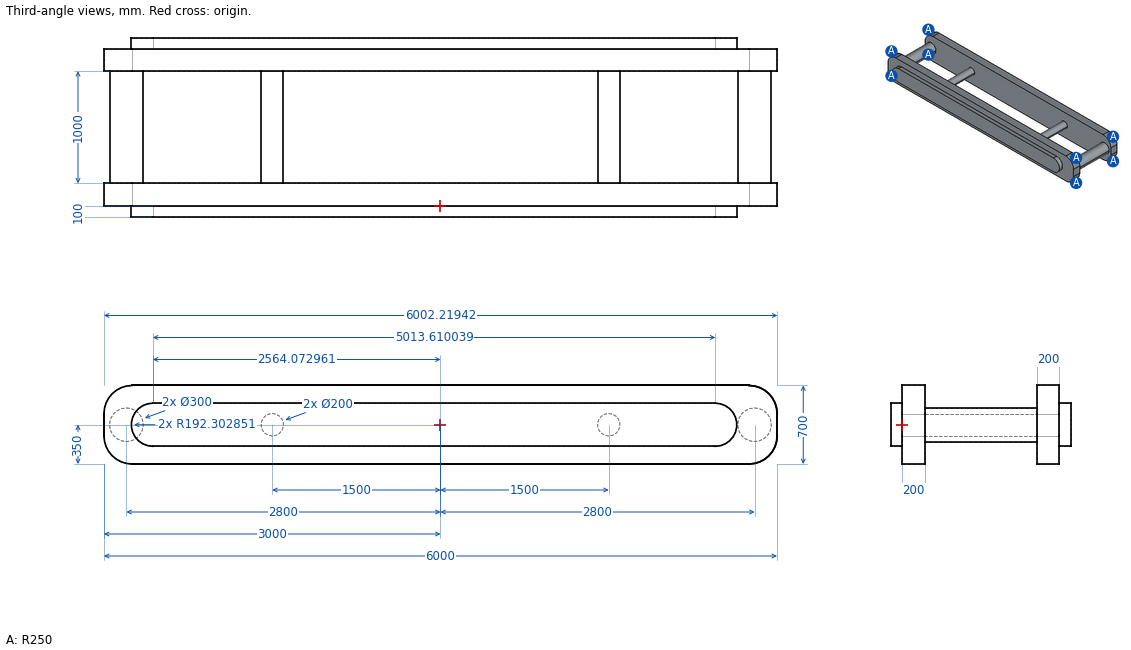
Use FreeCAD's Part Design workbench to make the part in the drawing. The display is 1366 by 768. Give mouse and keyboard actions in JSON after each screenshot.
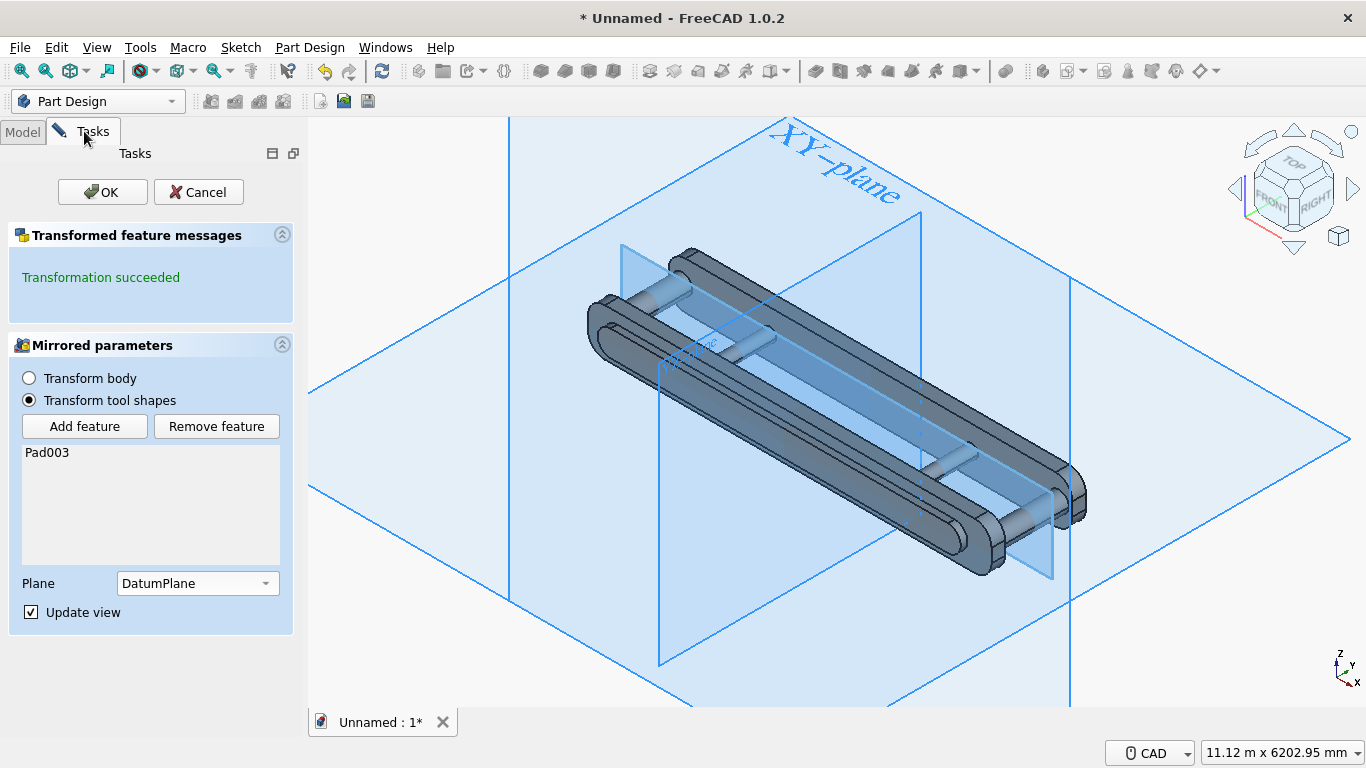
{"action": "left_click", "coordinate": [103, 192]}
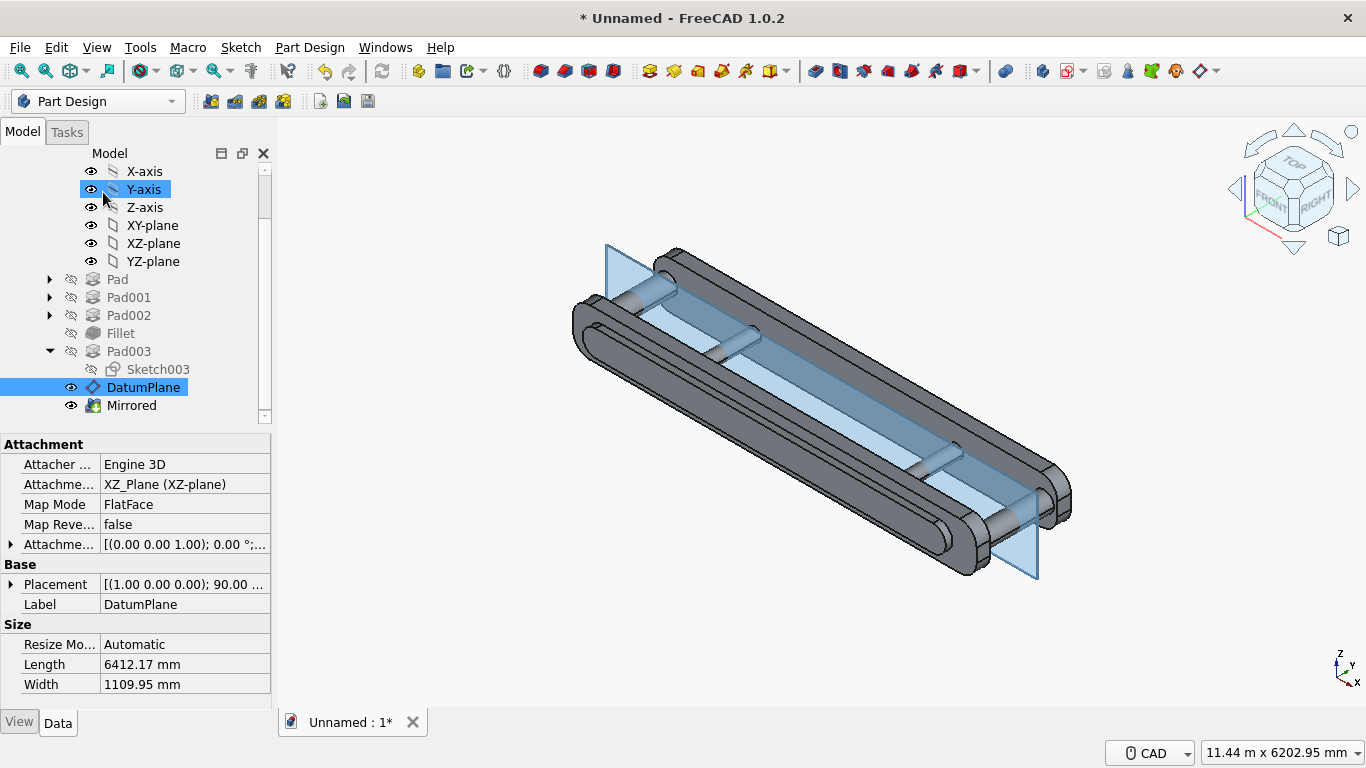
{"action": "left_click", "coordinate": [116, 387]}
{"action": "key", "text": "space"}